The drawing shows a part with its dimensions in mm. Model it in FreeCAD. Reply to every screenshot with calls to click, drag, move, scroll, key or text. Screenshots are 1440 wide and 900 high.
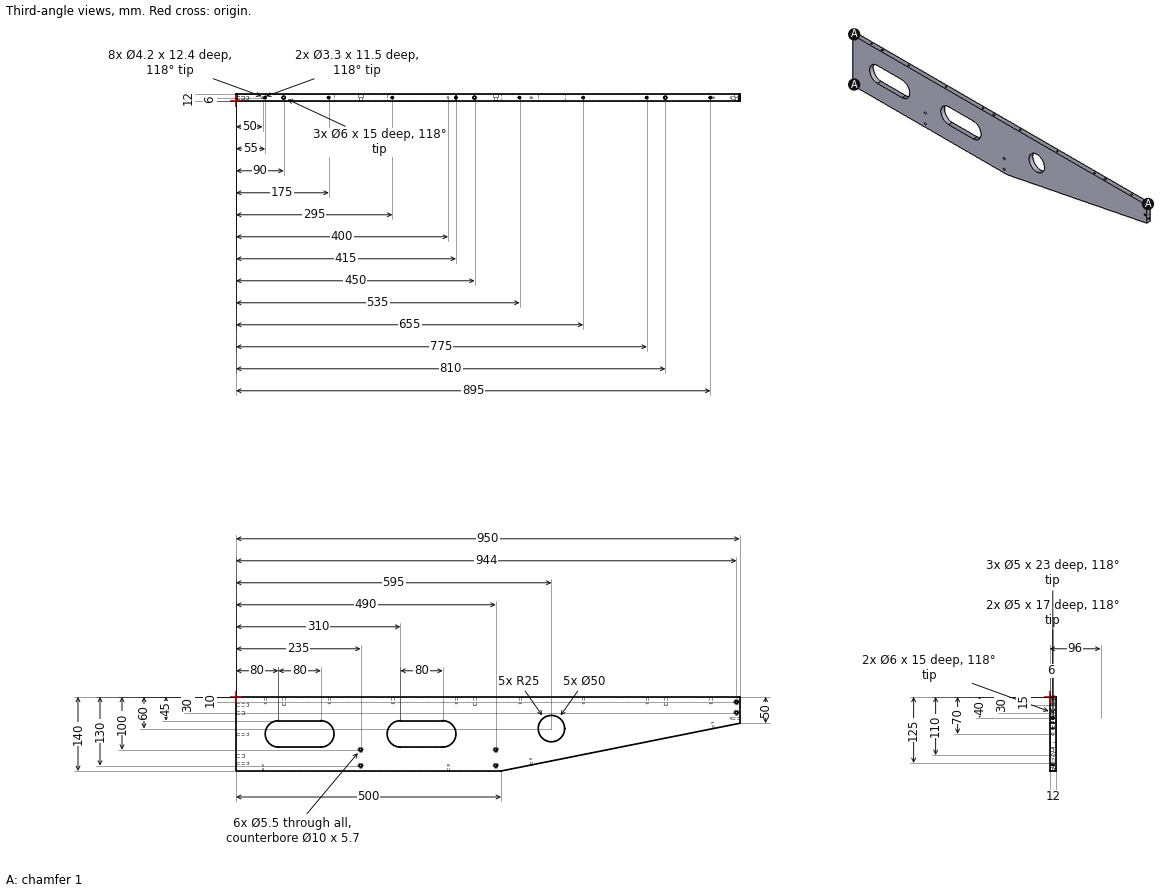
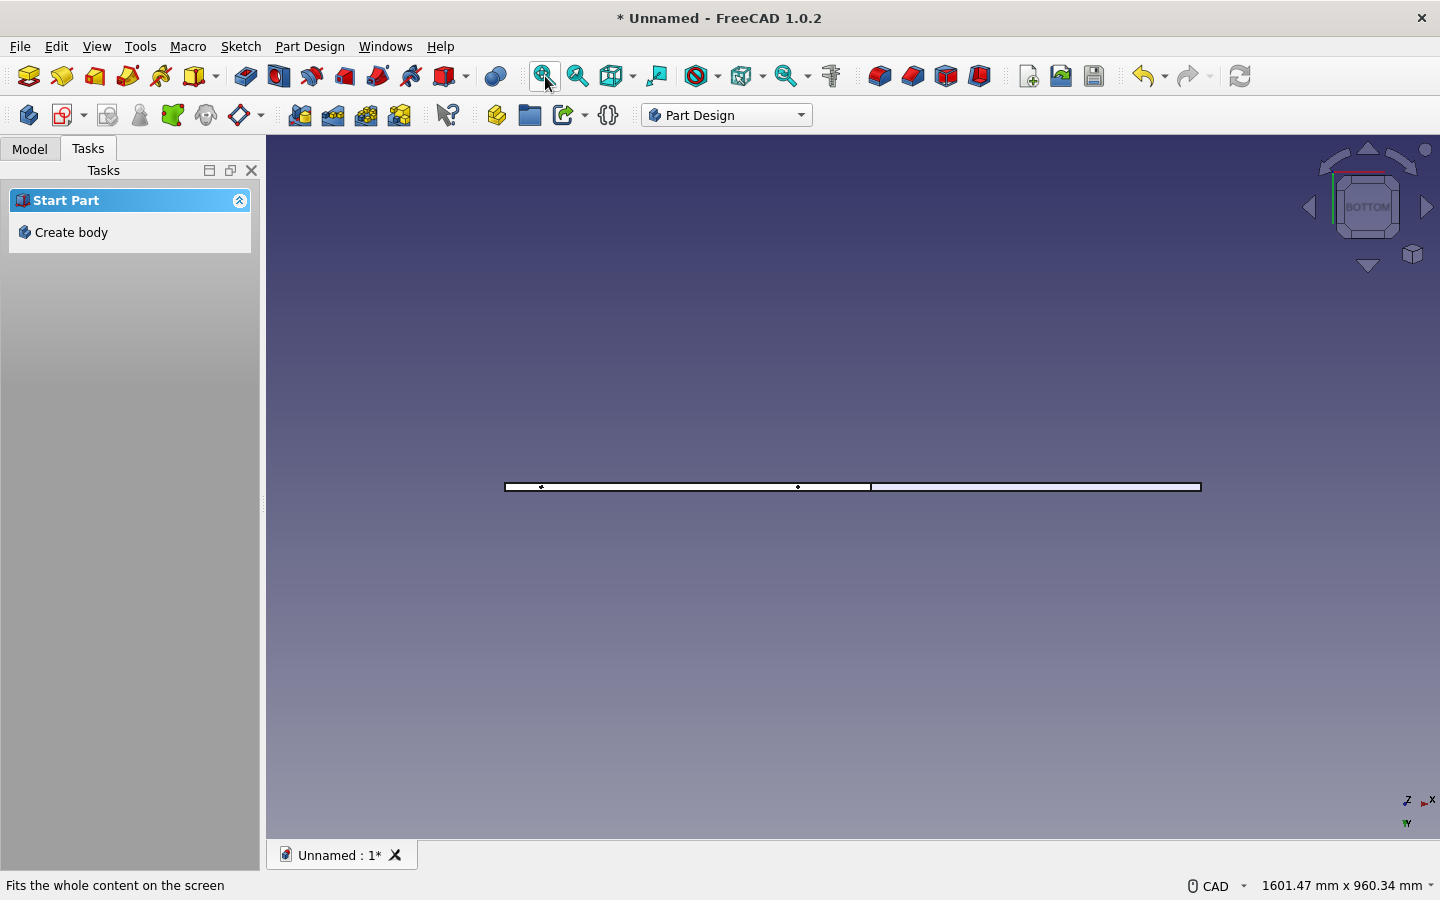
scroll(1131, 486, up, 6)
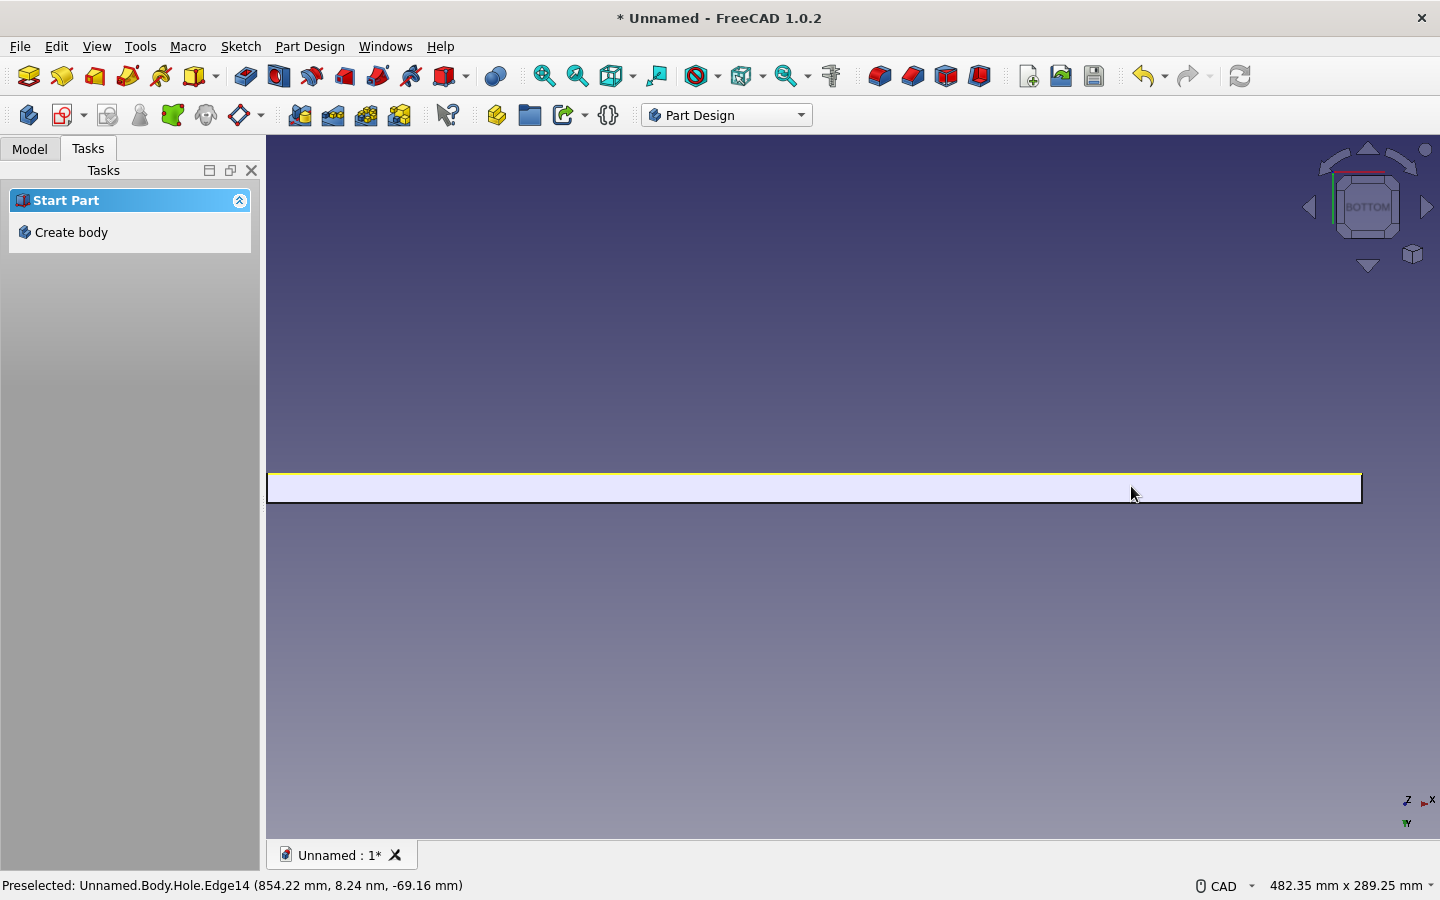
click(1128, 487)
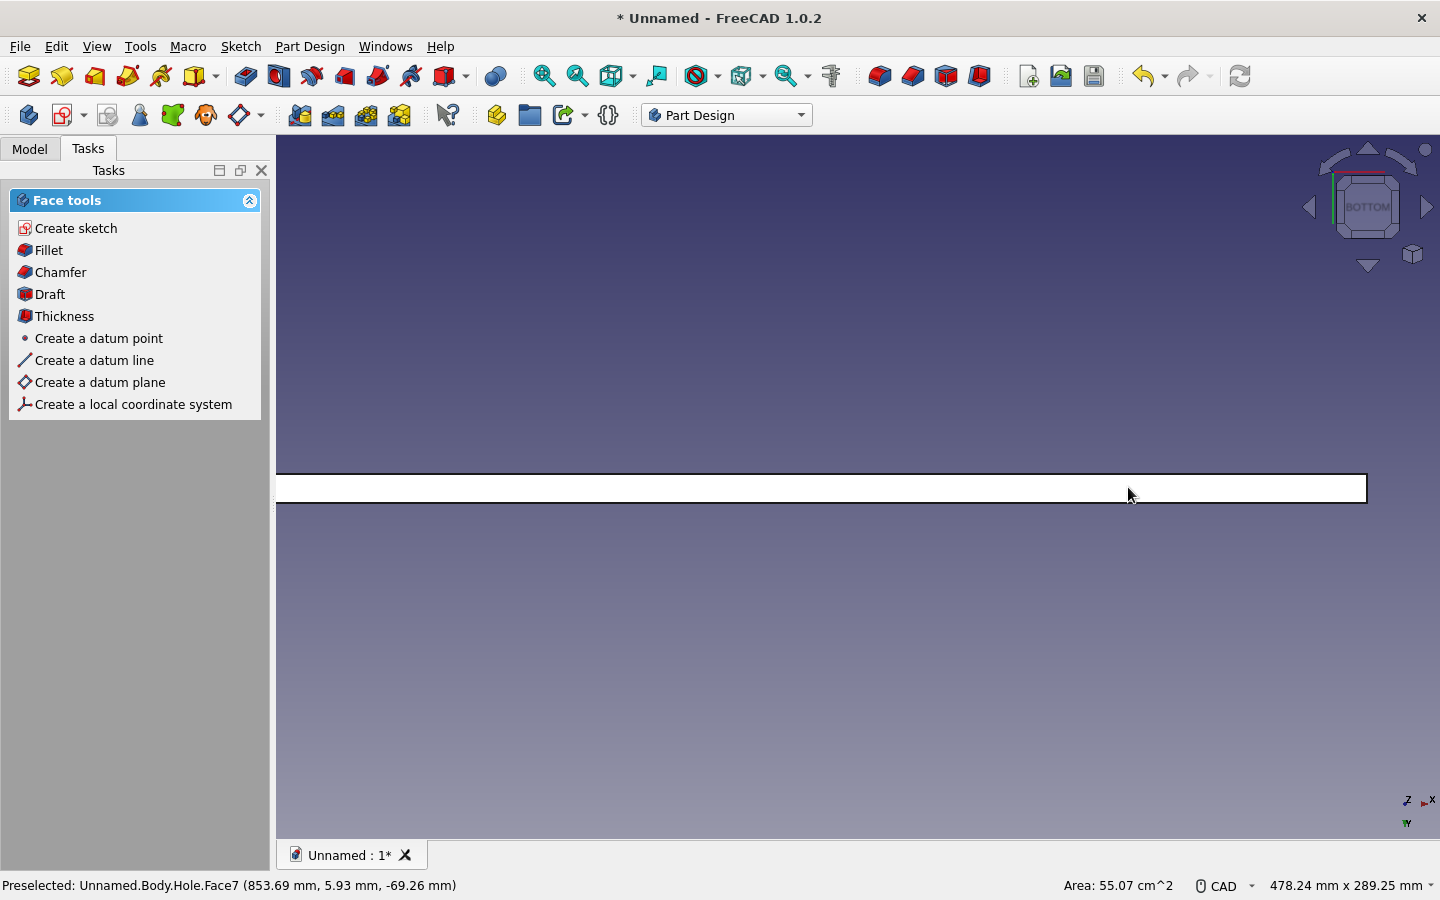
click(62, 116)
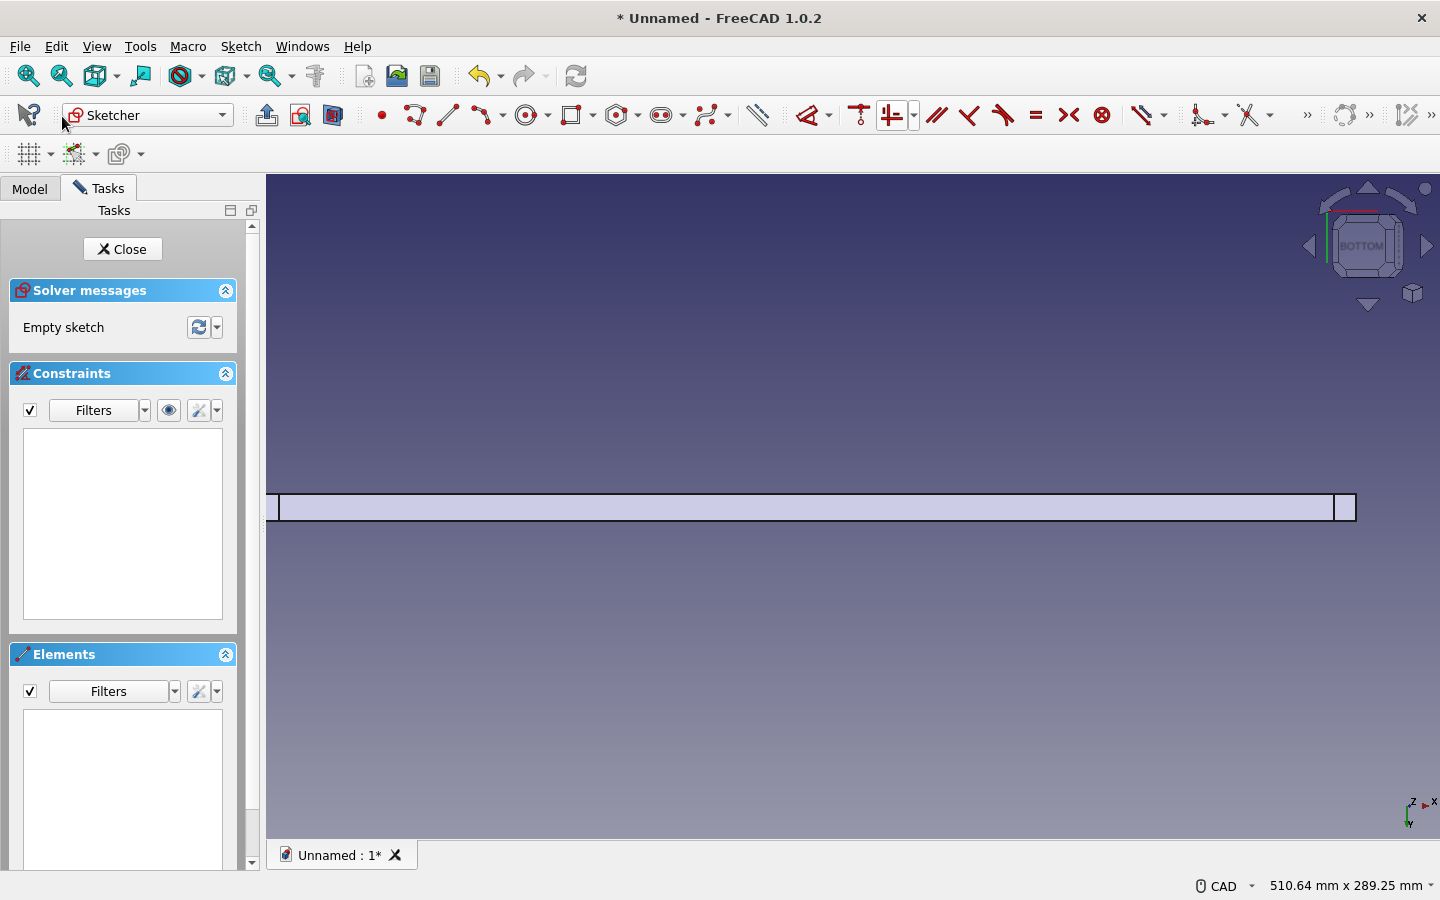
key(q)
key(s)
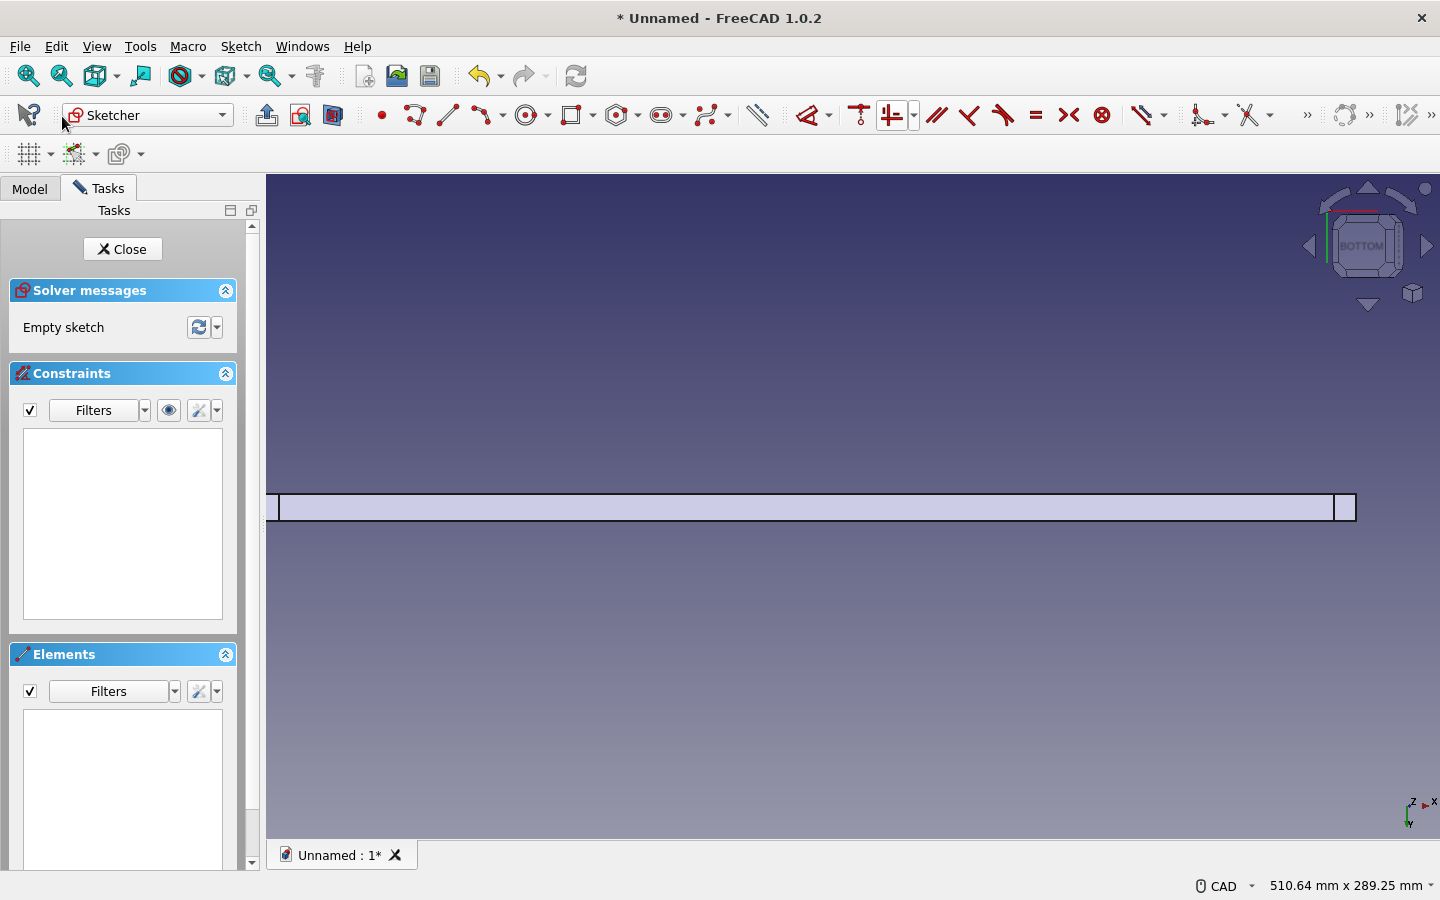
scroll(1114, 509, down, 5)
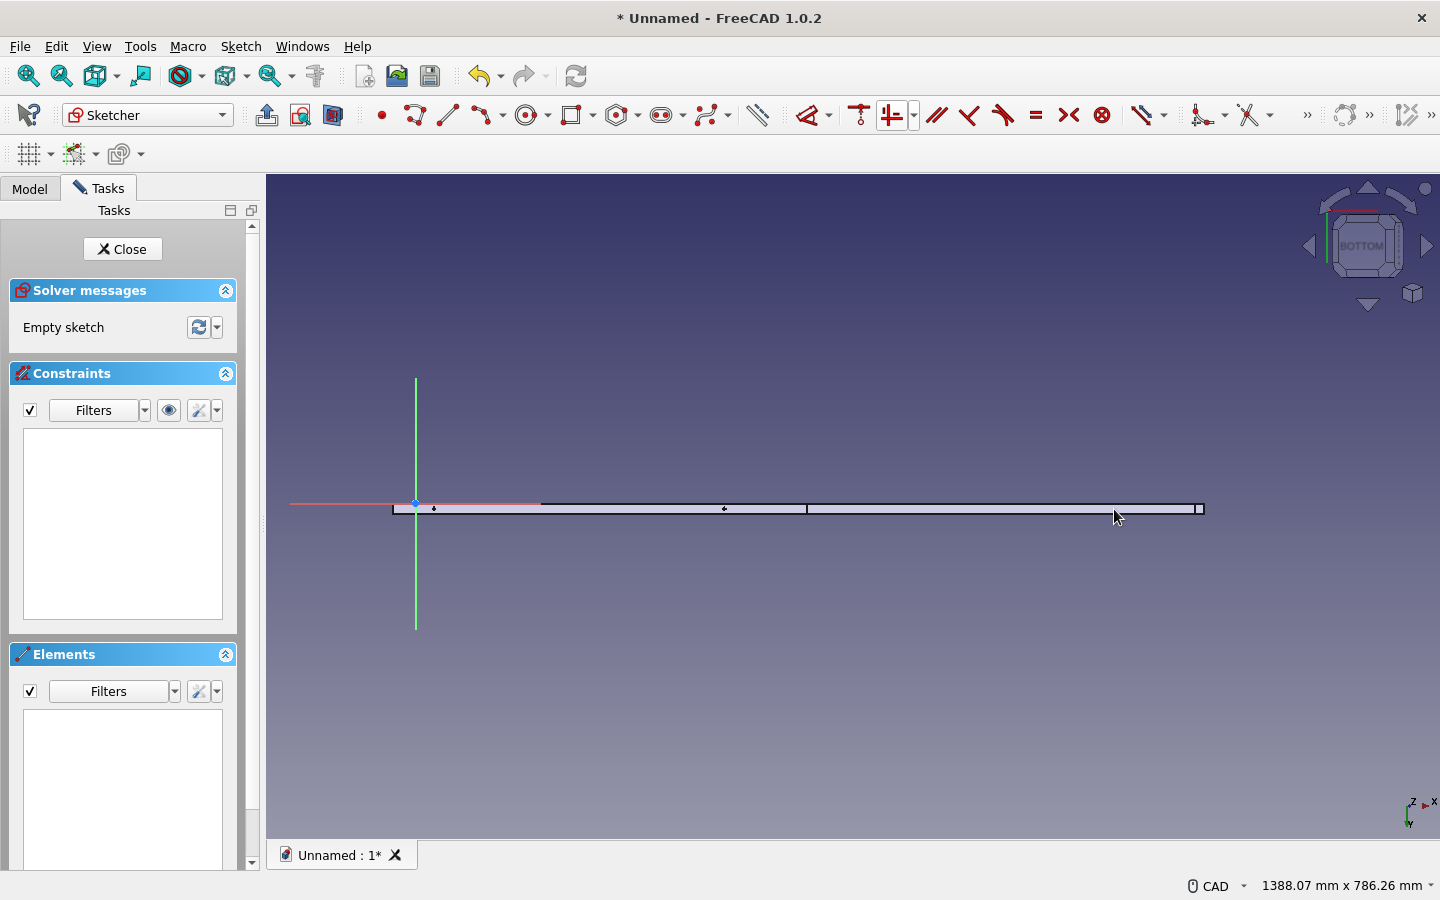
click(526, 116)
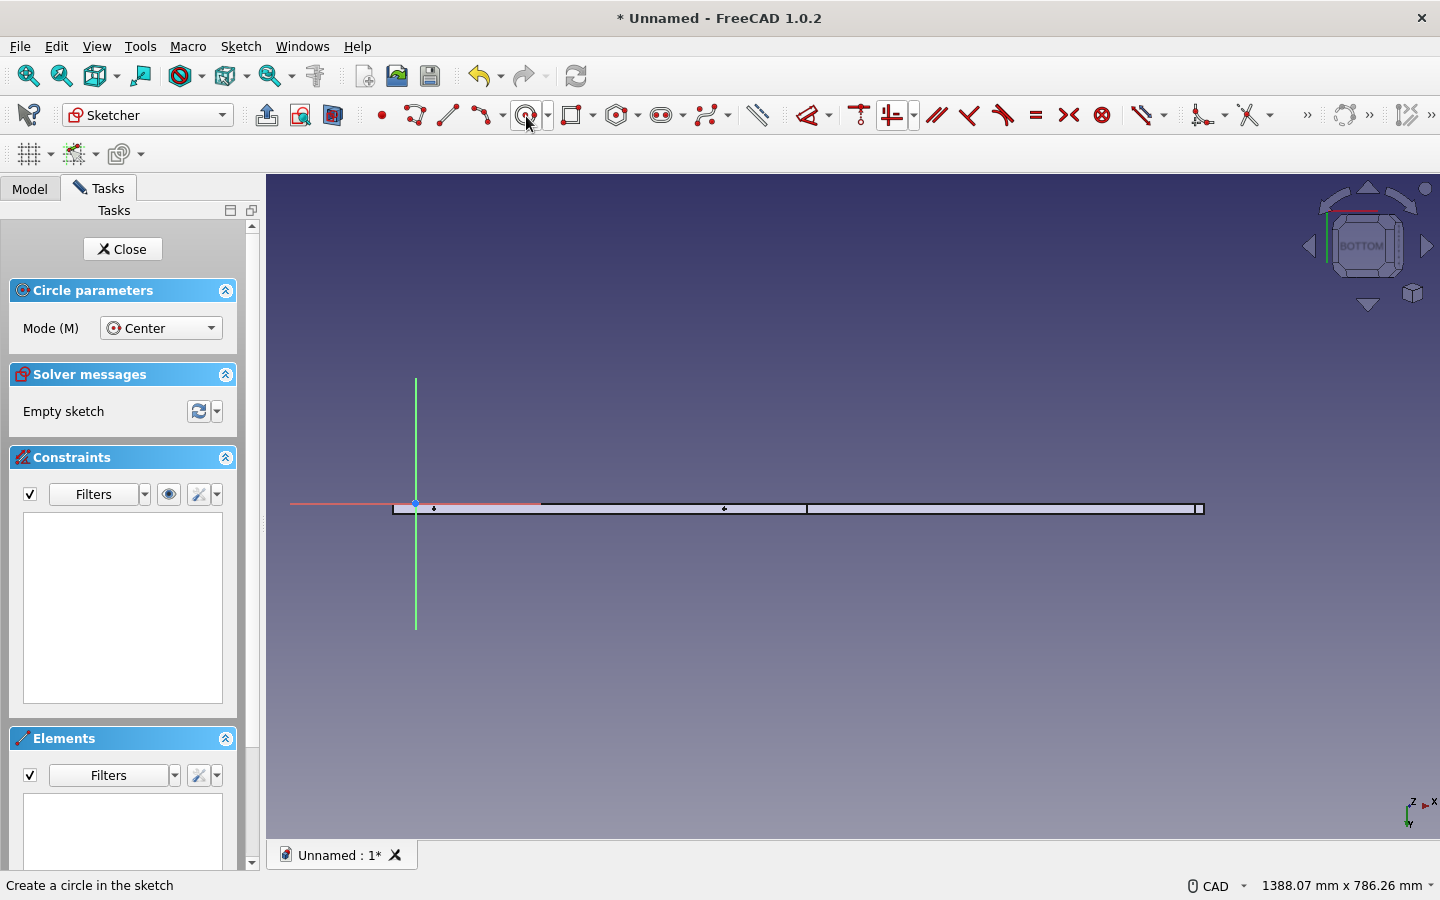
scroll(1153, 509, up, 14)